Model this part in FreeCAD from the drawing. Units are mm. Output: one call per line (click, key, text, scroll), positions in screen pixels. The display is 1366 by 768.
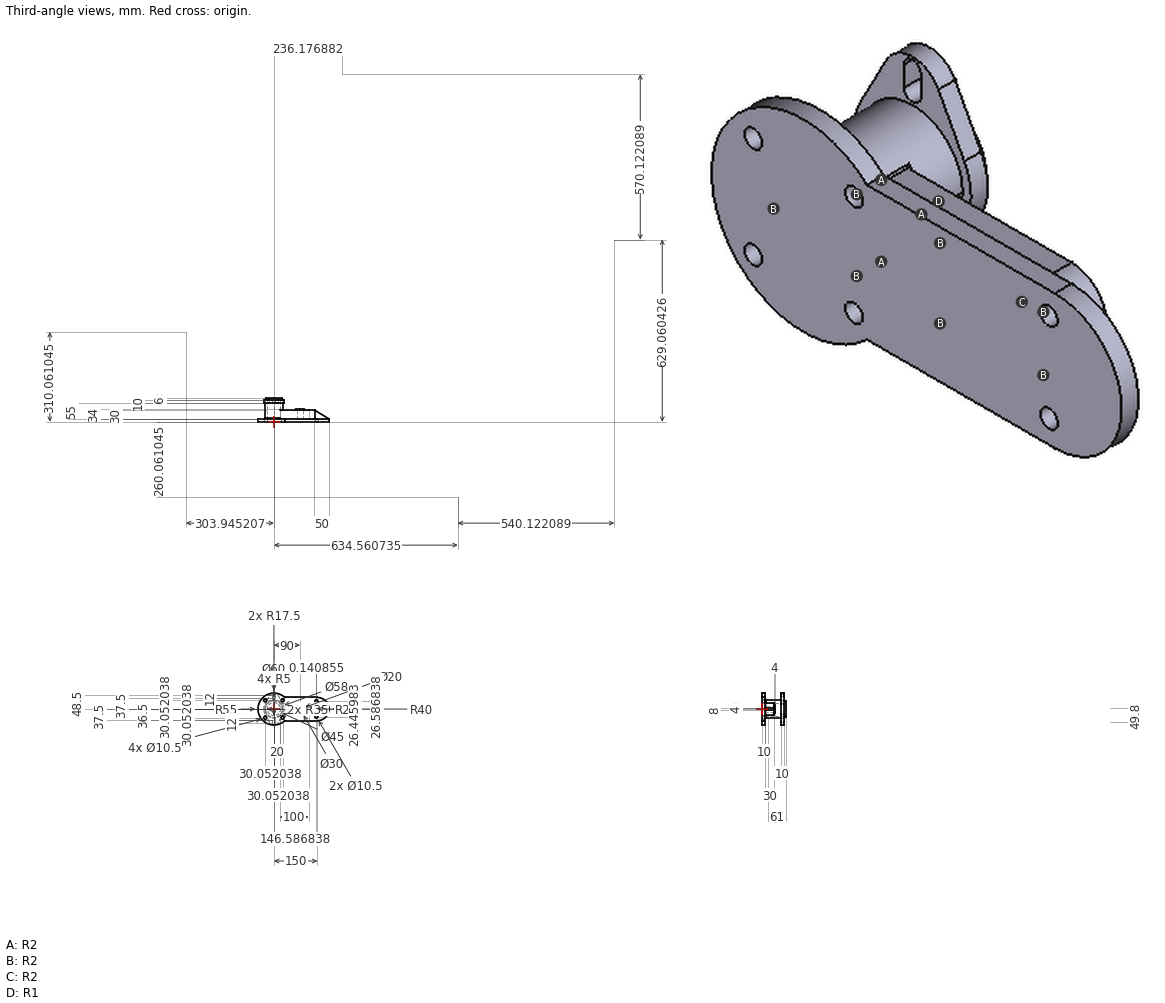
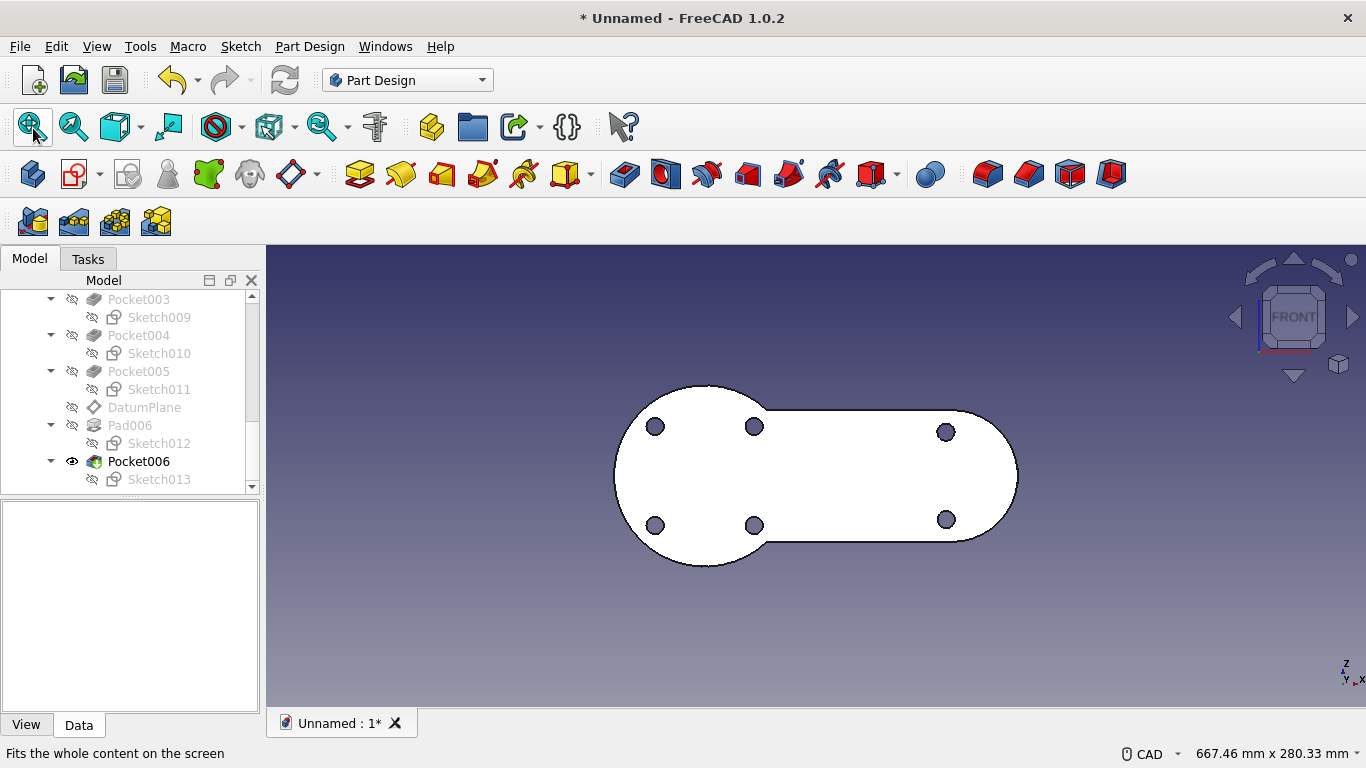
key(3)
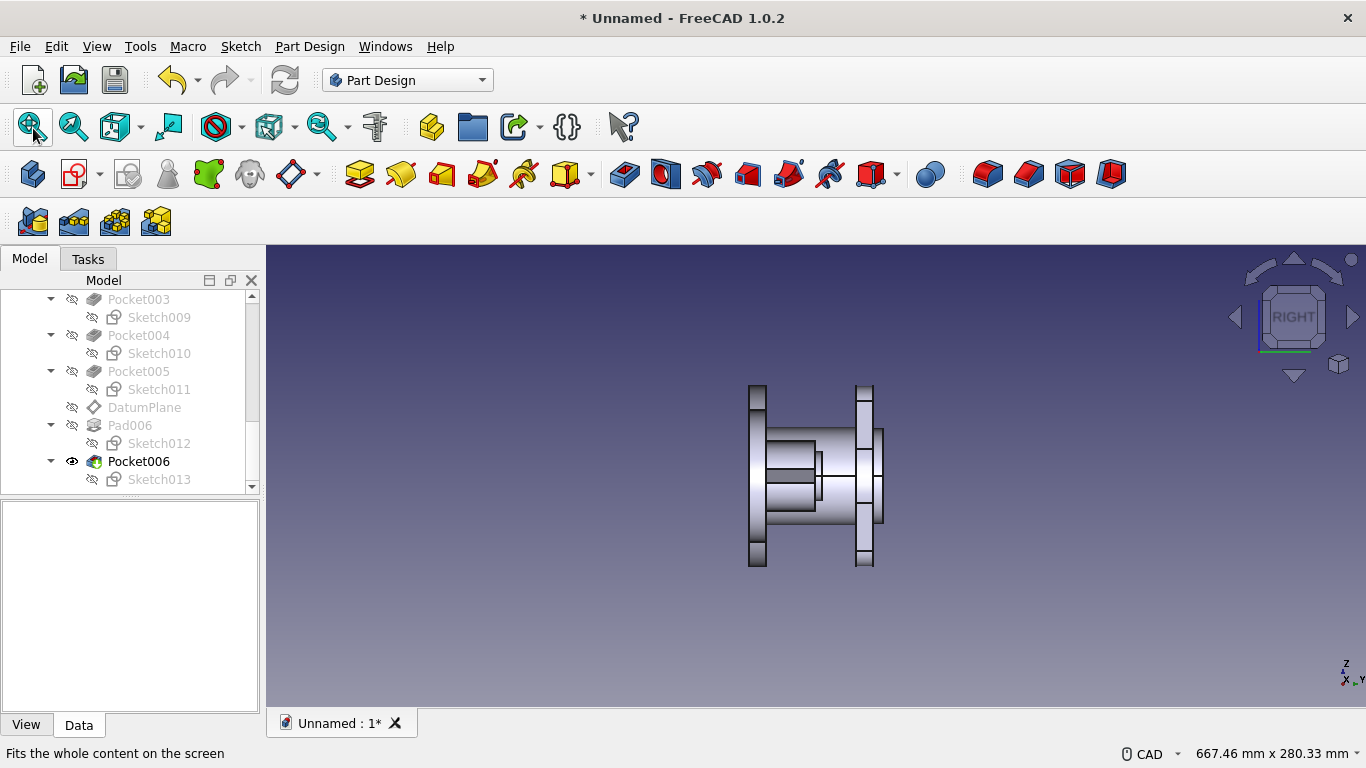
click(33, 128)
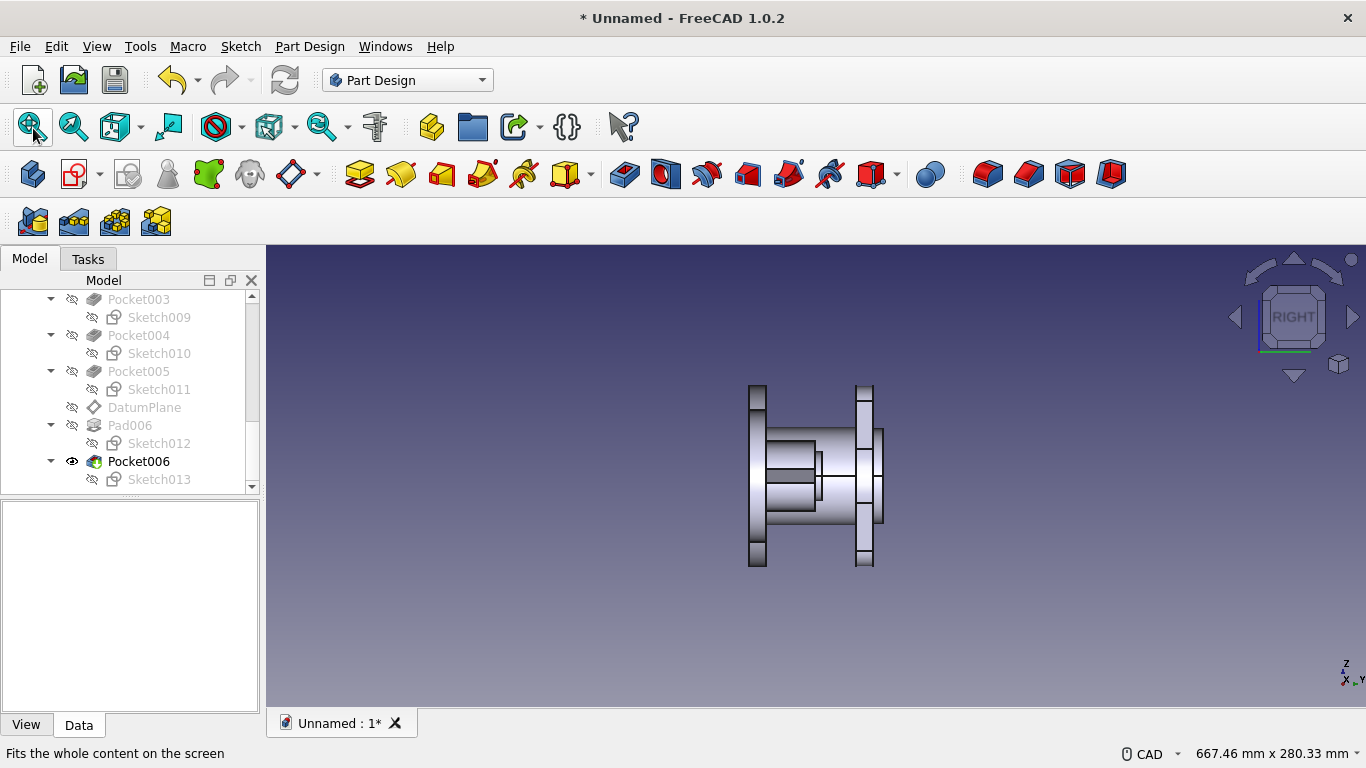
key(5)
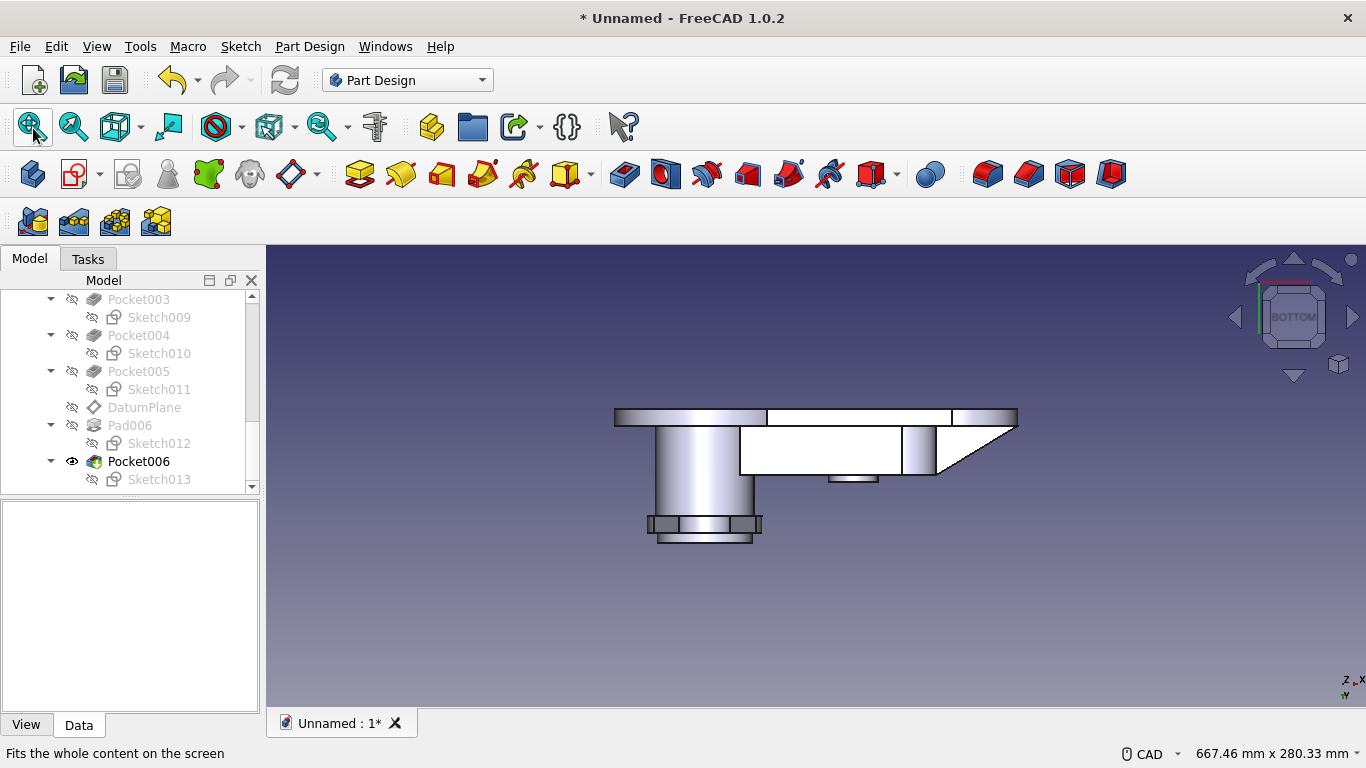
key(v)
key(f)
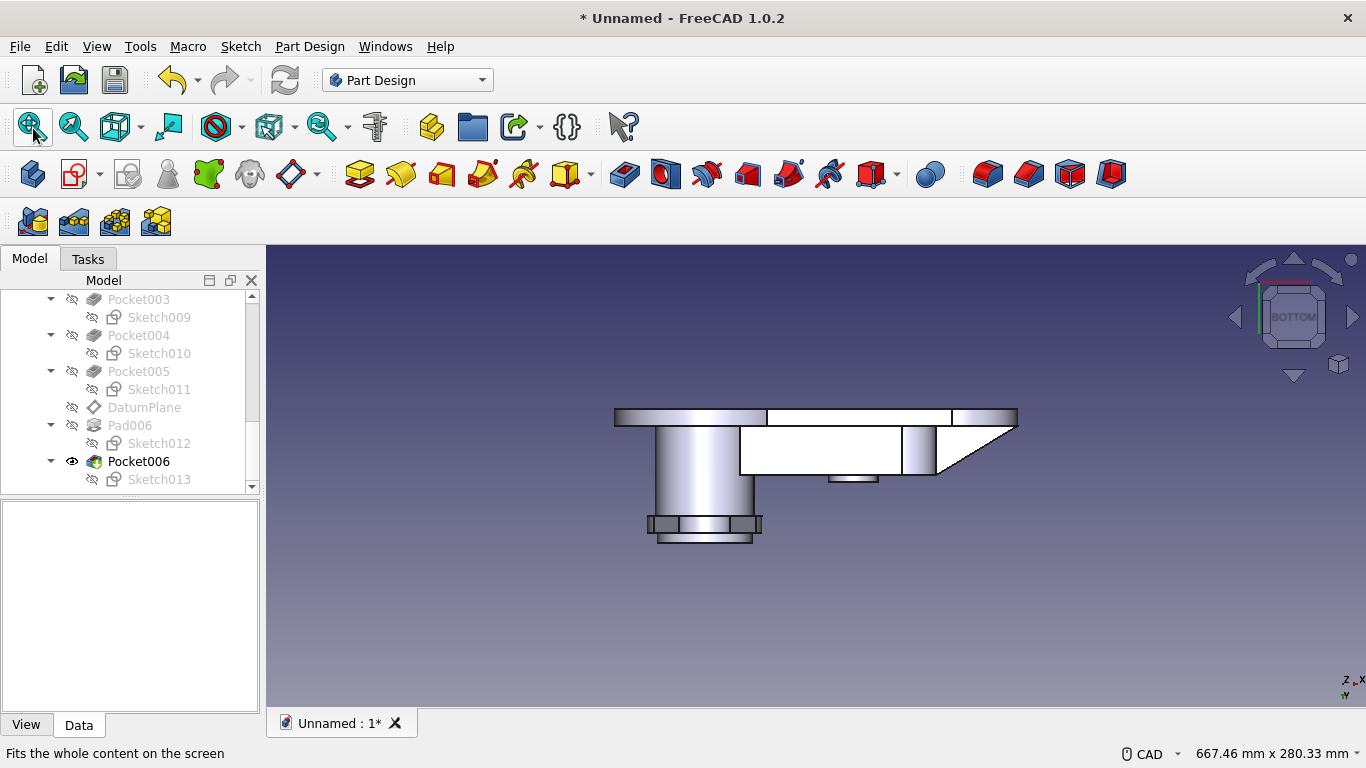
key(4)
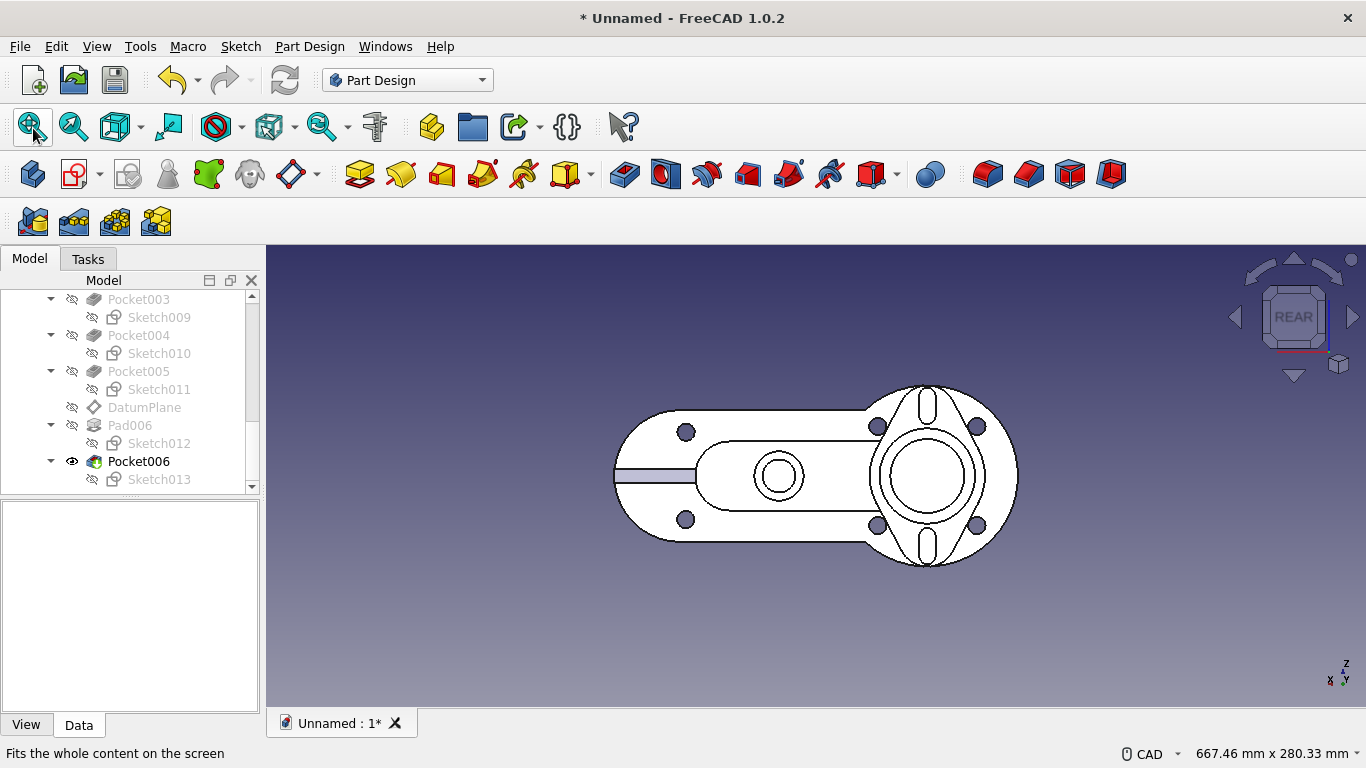
key(v)
key(f)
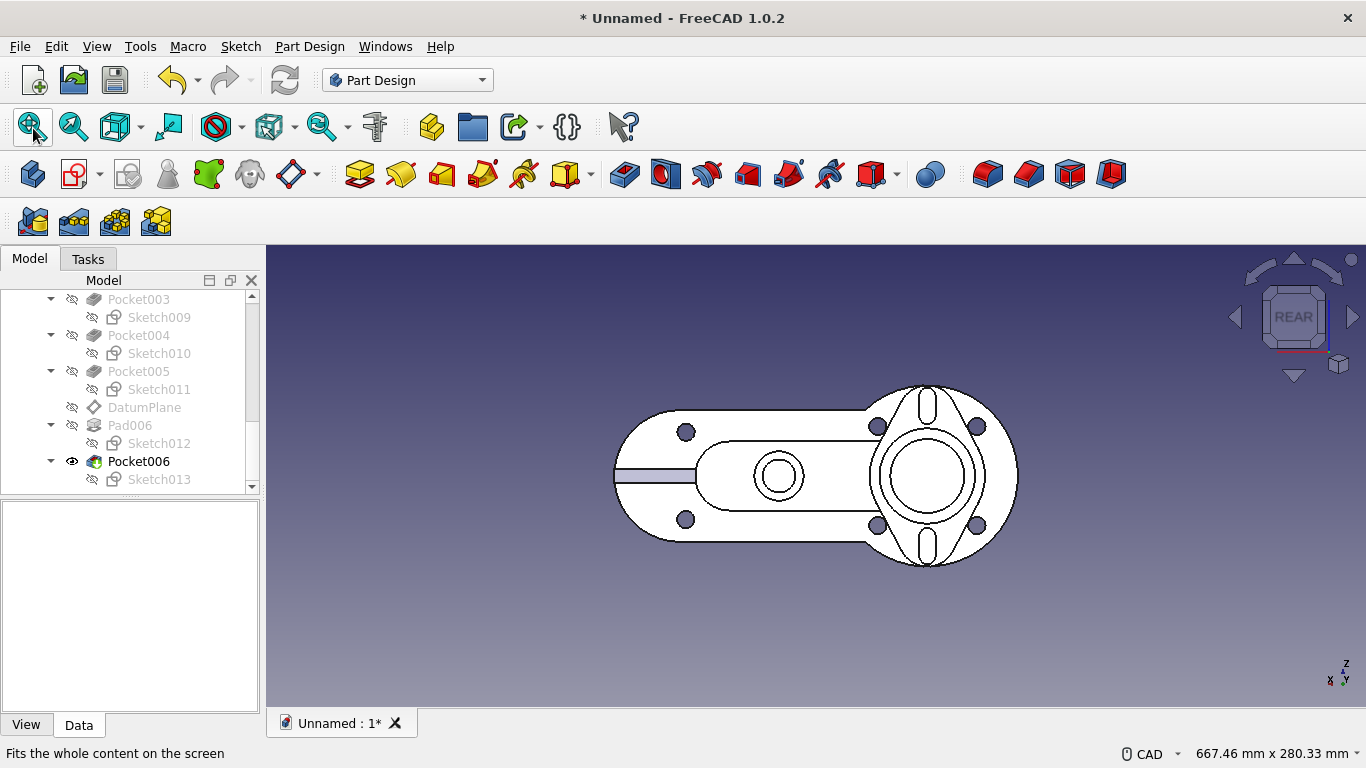
key(6)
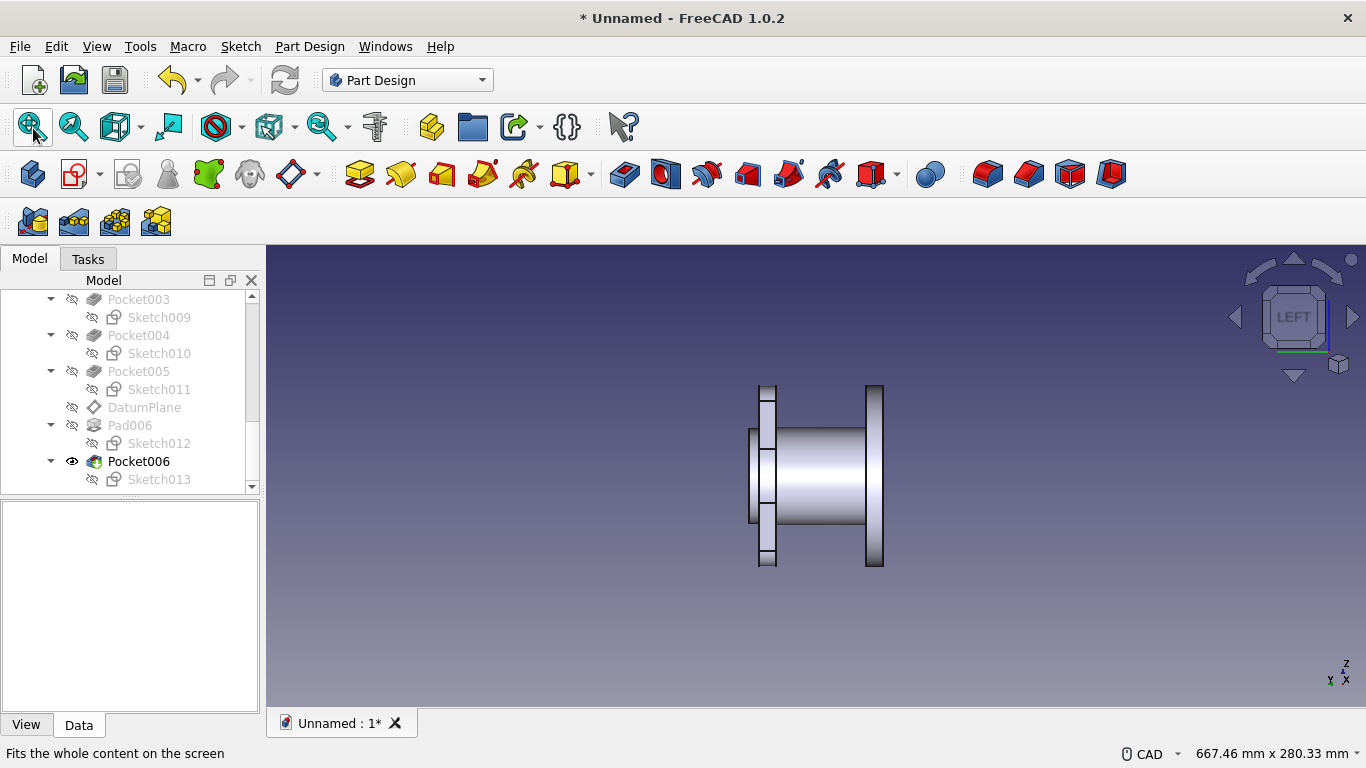
key(v)
key(f)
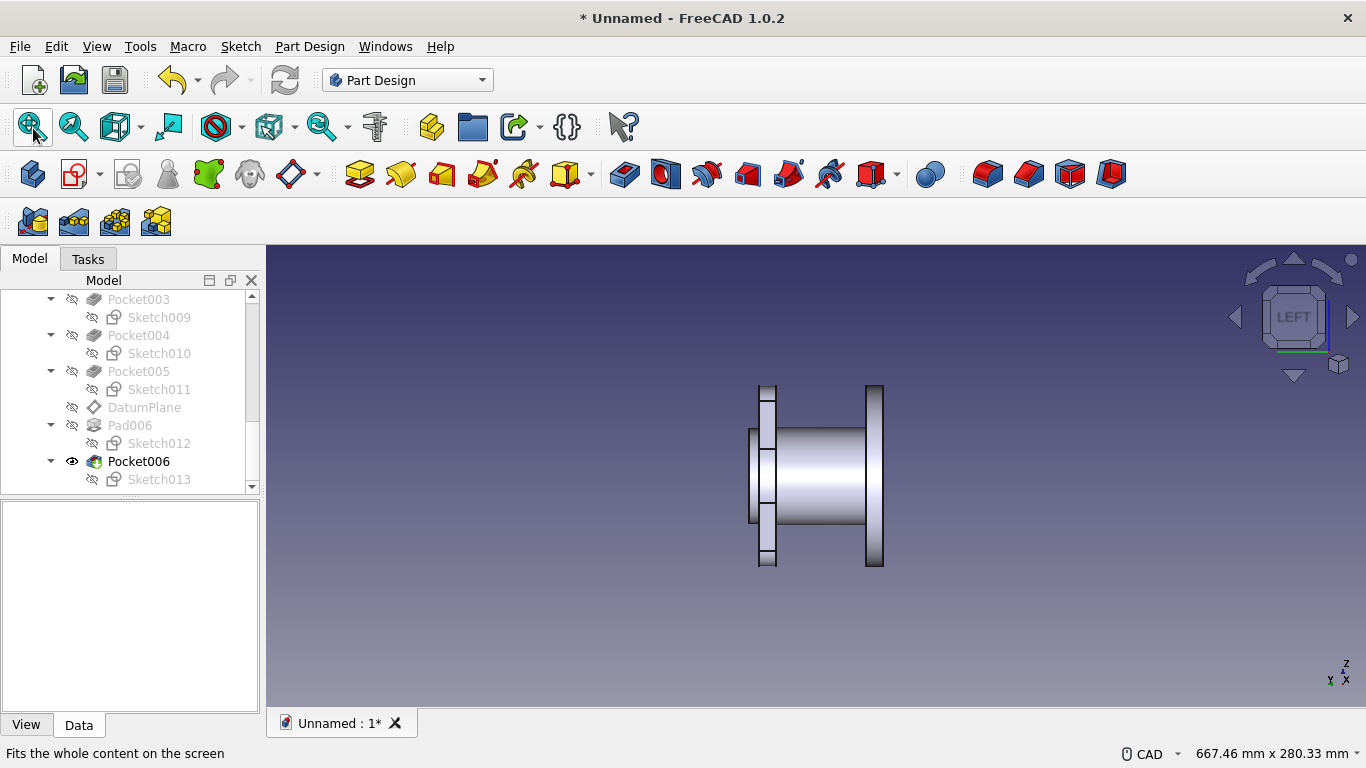
key(v)
key(3)